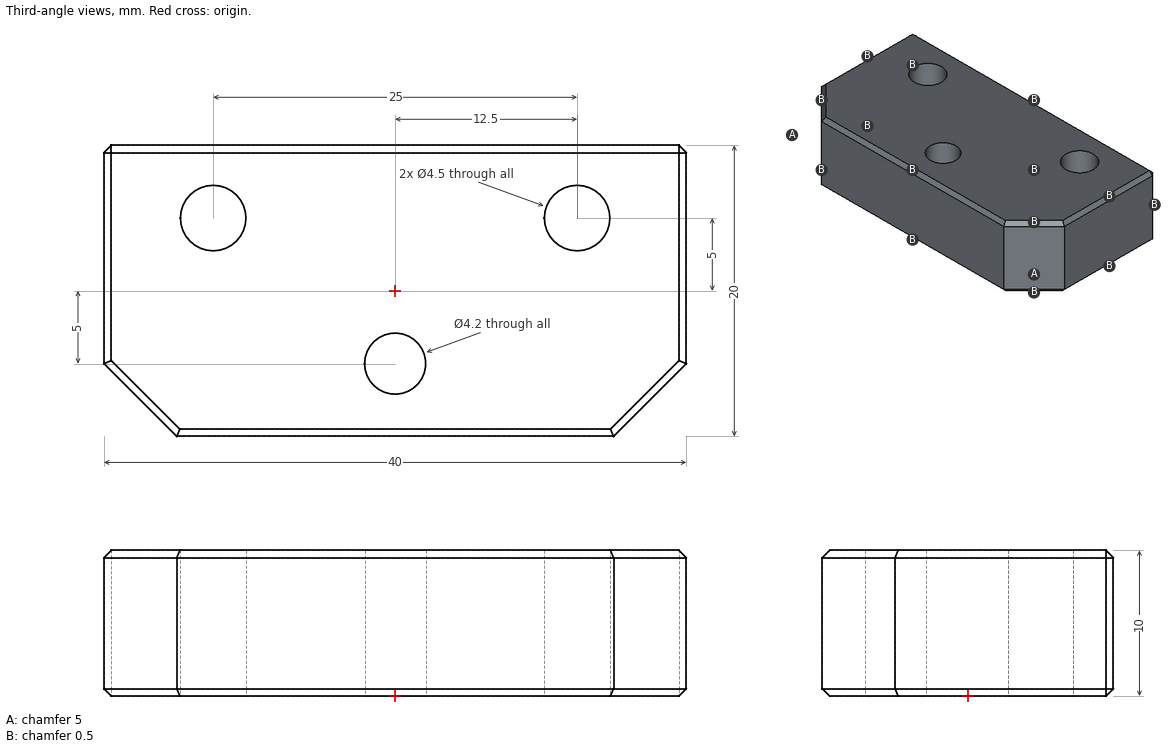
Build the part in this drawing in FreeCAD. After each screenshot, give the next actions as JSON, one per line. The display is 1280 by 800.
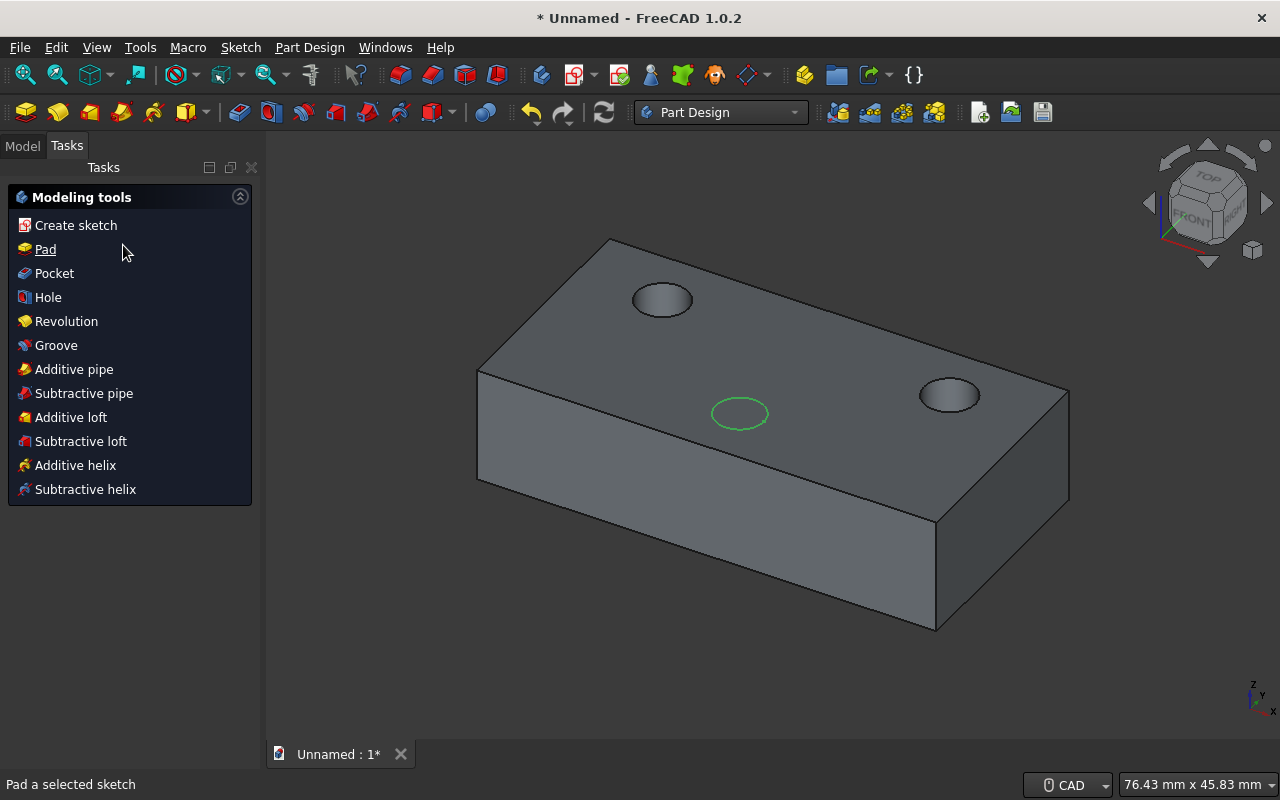
{"action": "left_click", "coordinate": [272, 112]}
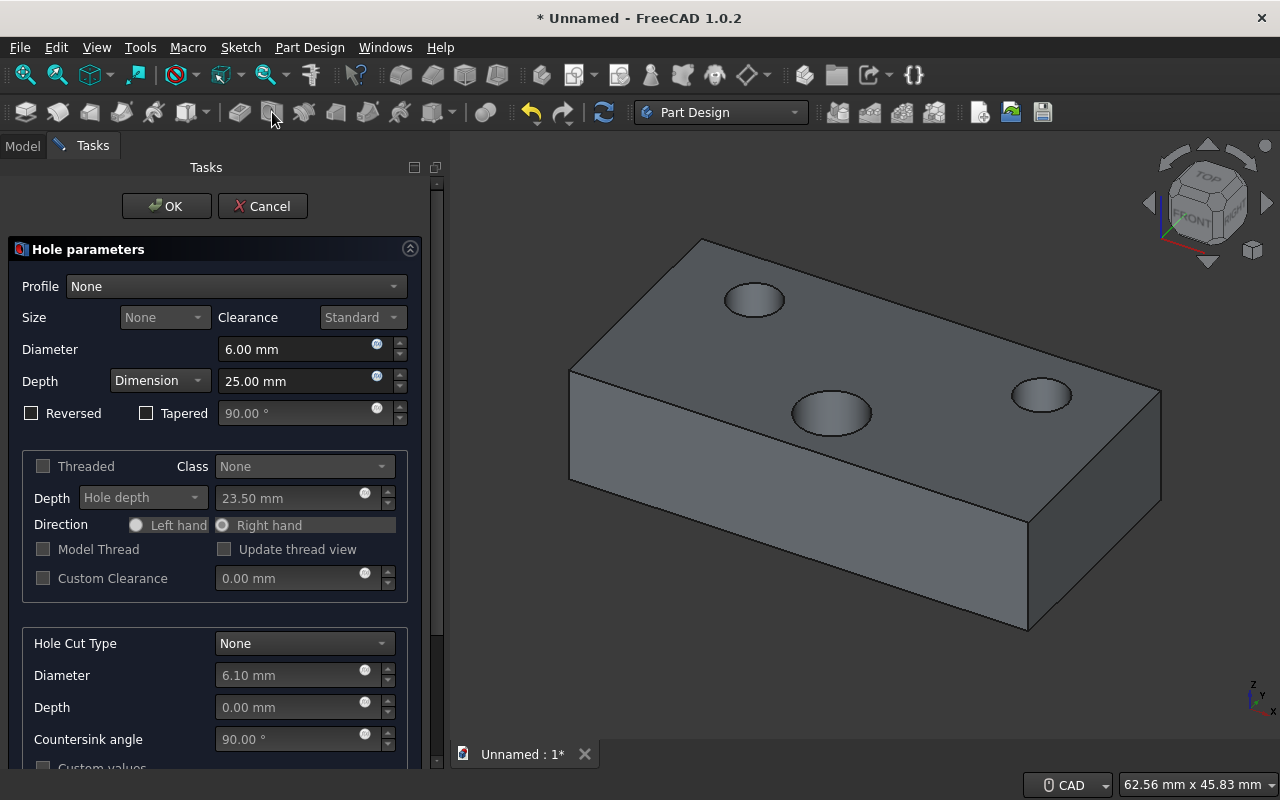
{"action": "triple_click", "coordinate": [305, 349]}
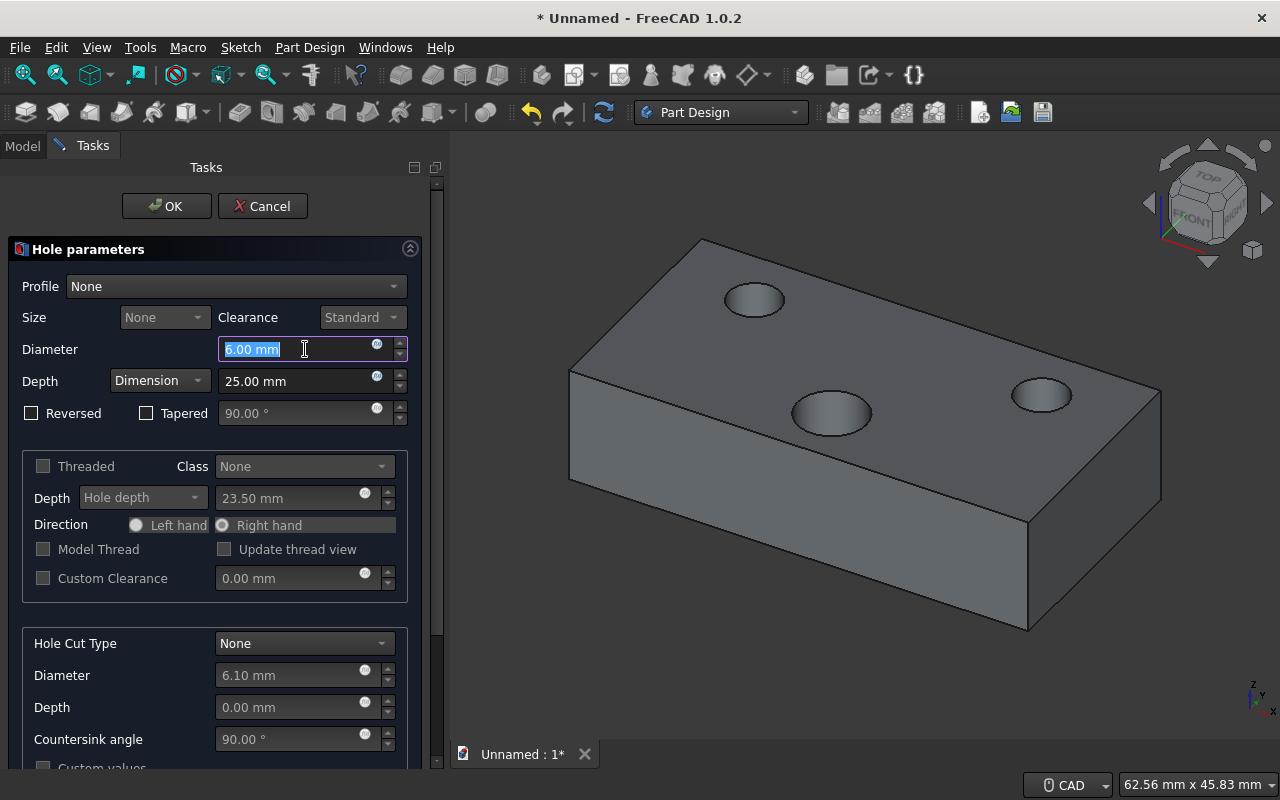
{"action": "type", "text": "4.2"}
{"action": "key", "text": "Tab"}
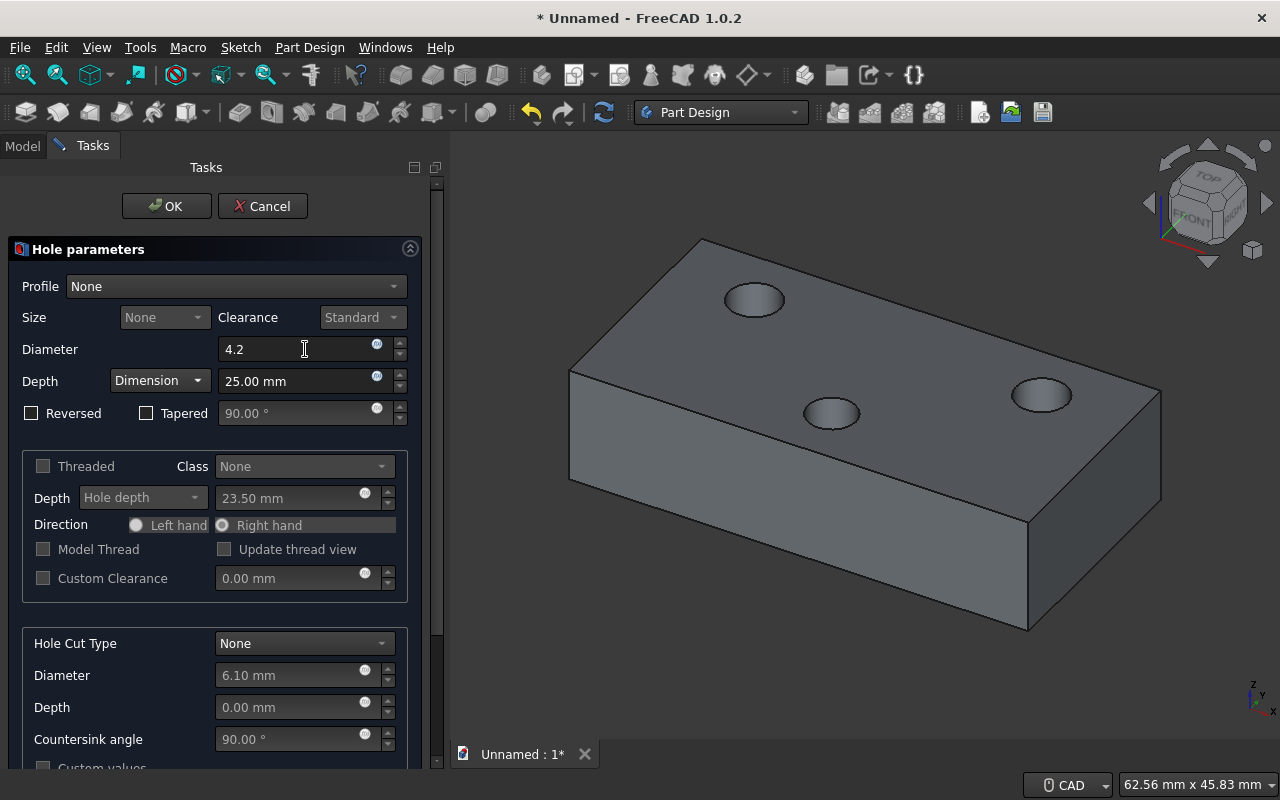
{"action": "left_click", "coordinate": [161, 380]}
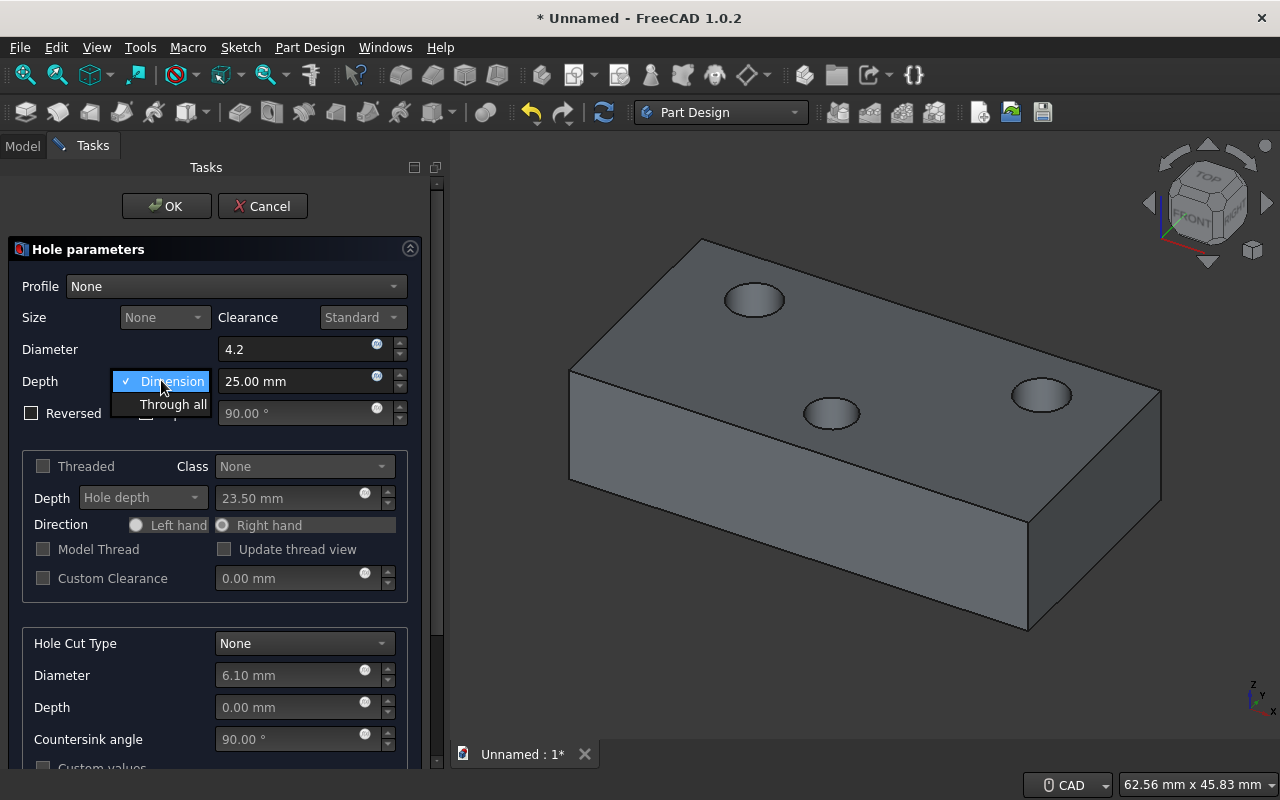
{"action": "left_click", "coordinate": [160, 404]}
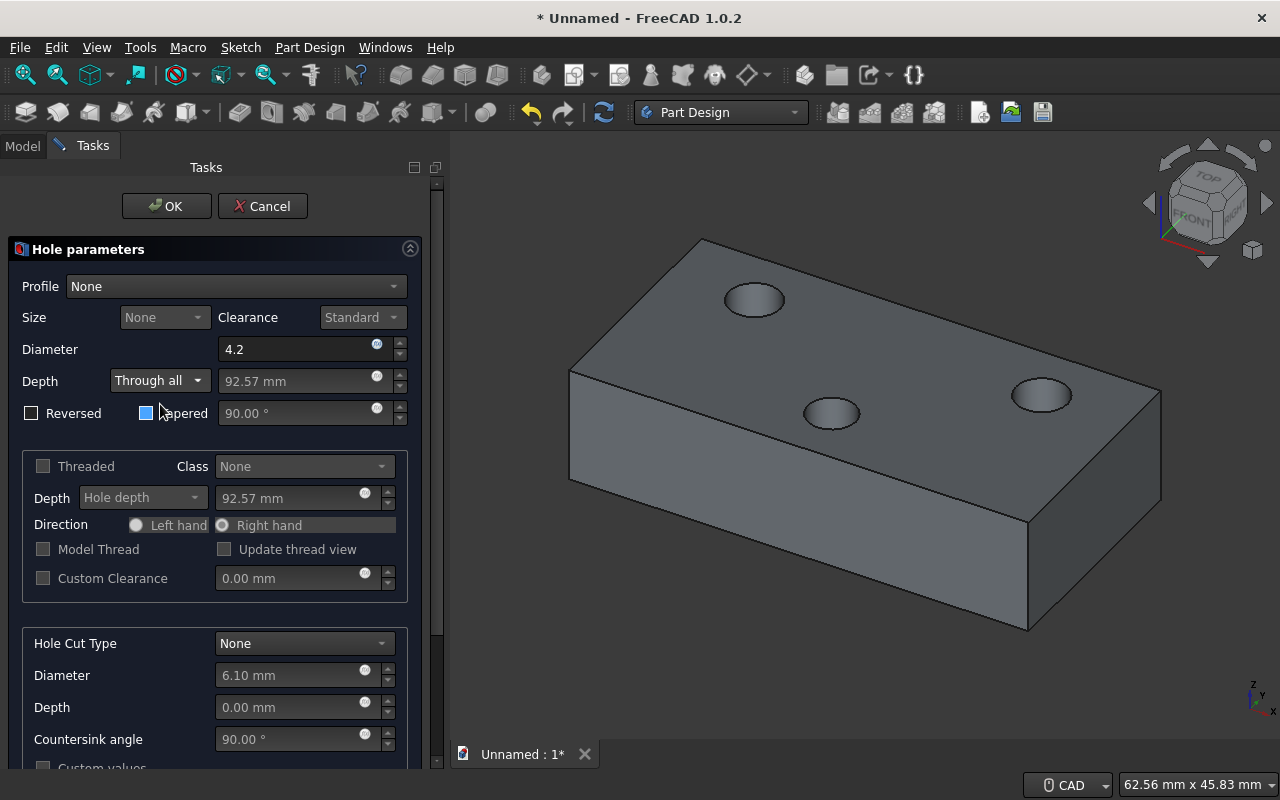
{"action": "left_click", "coordinate": [167, 206]}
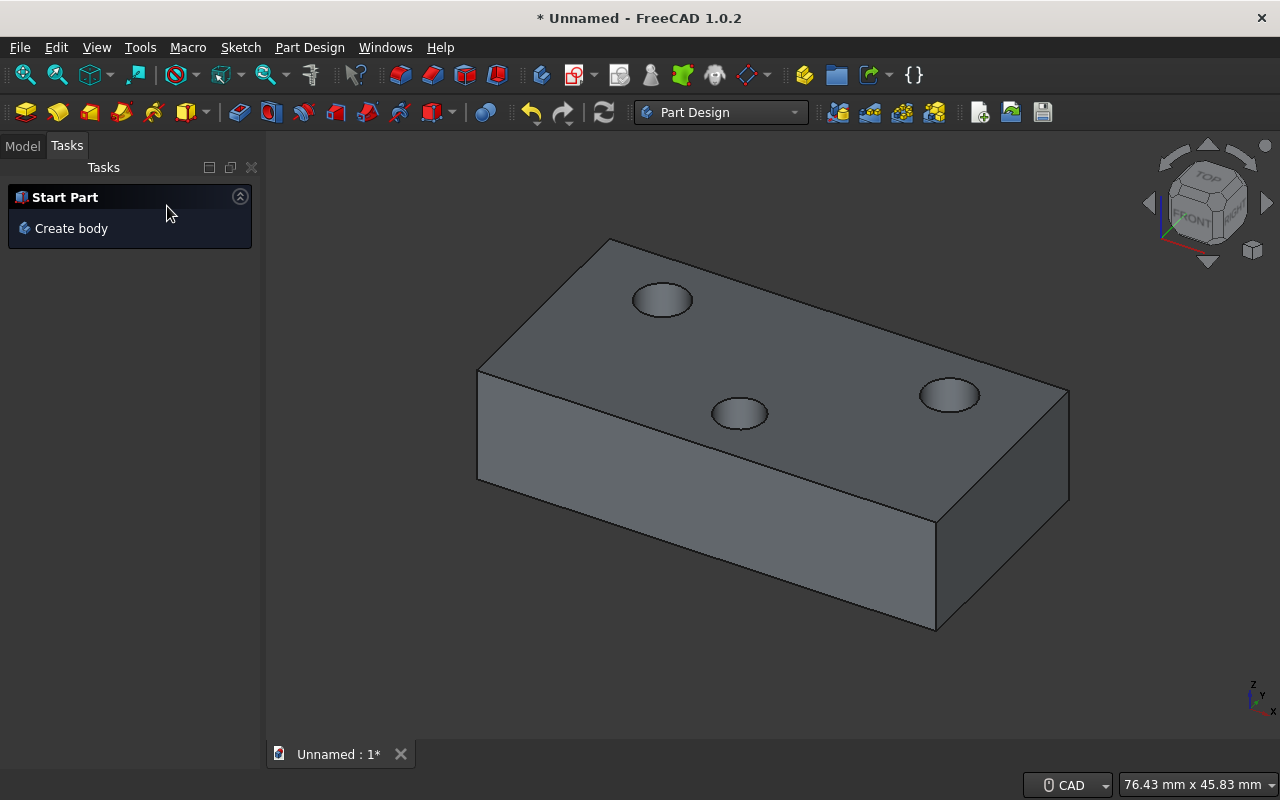
{"action": "left_click", "coordinate": [936, 576]}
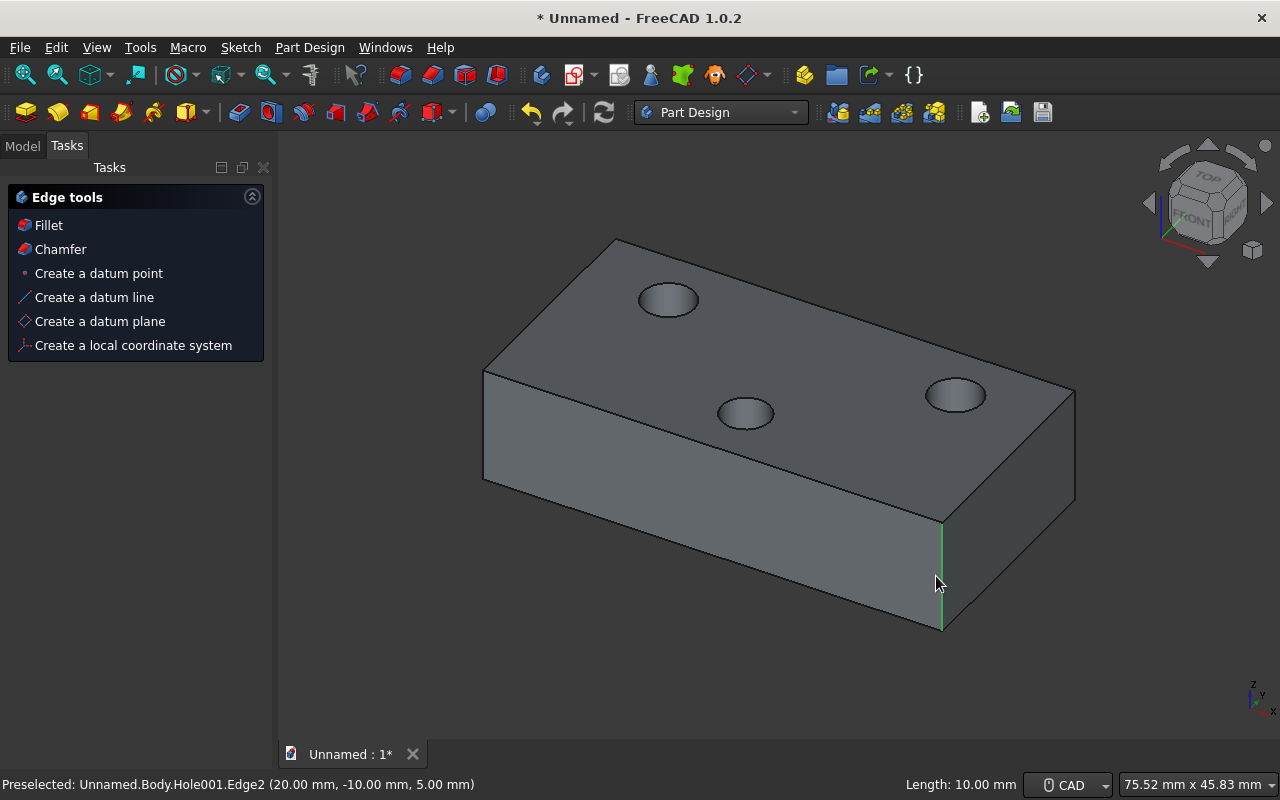
{"action": "key", "text": "0"}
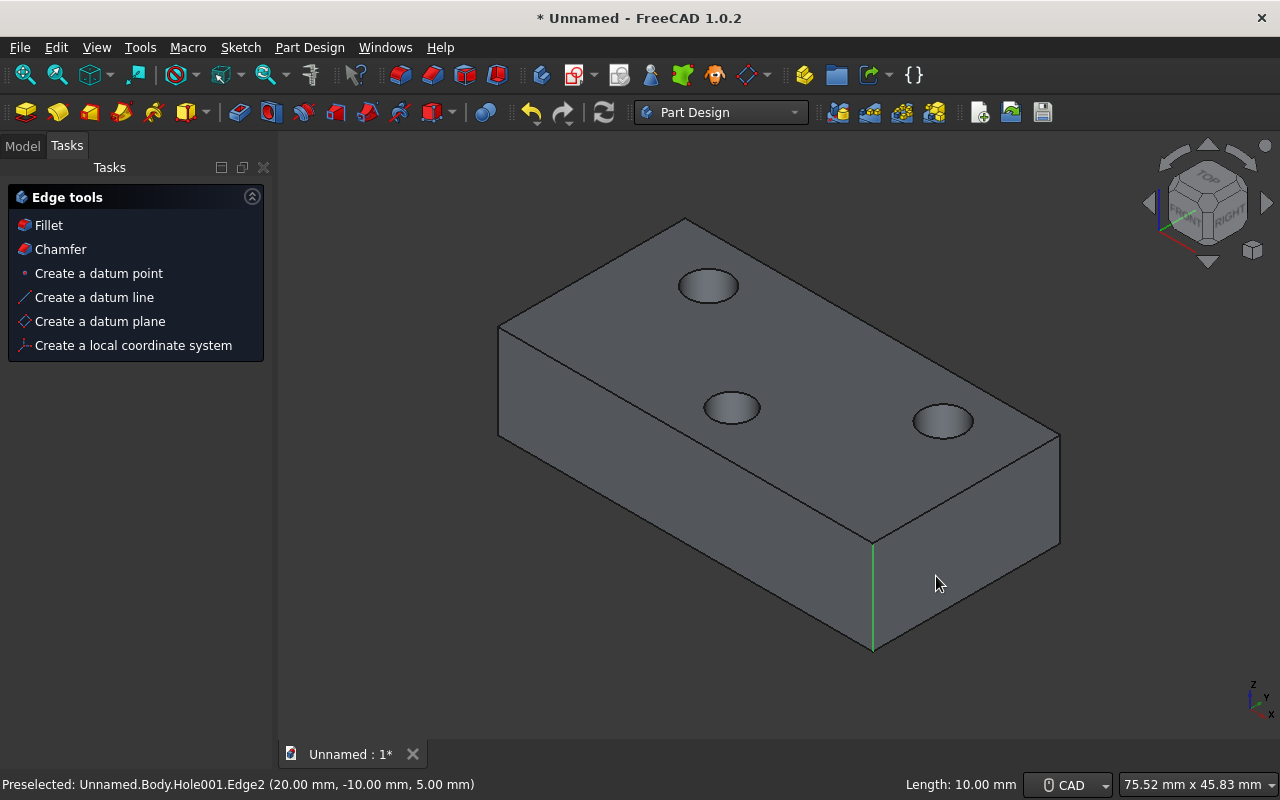
{"action": "key", "text": "2"}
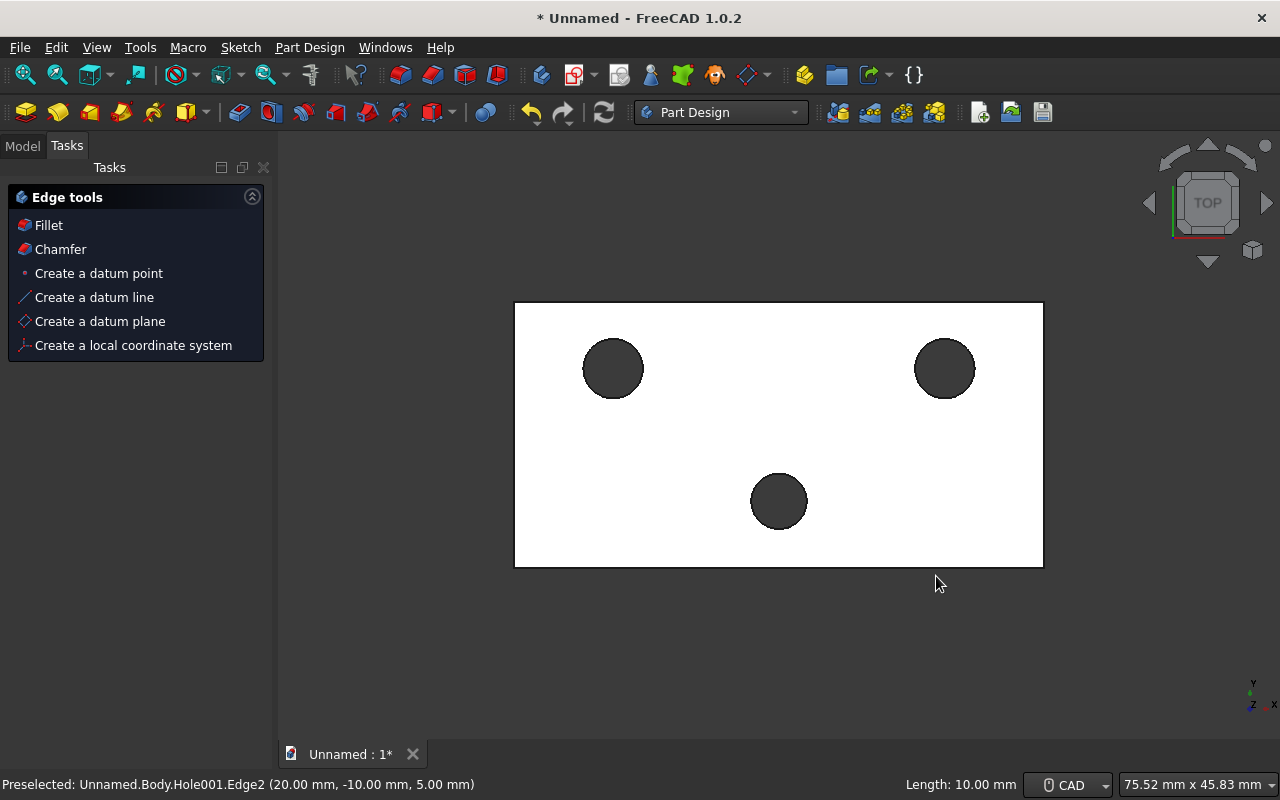
{"action": "key", "text": "1"}